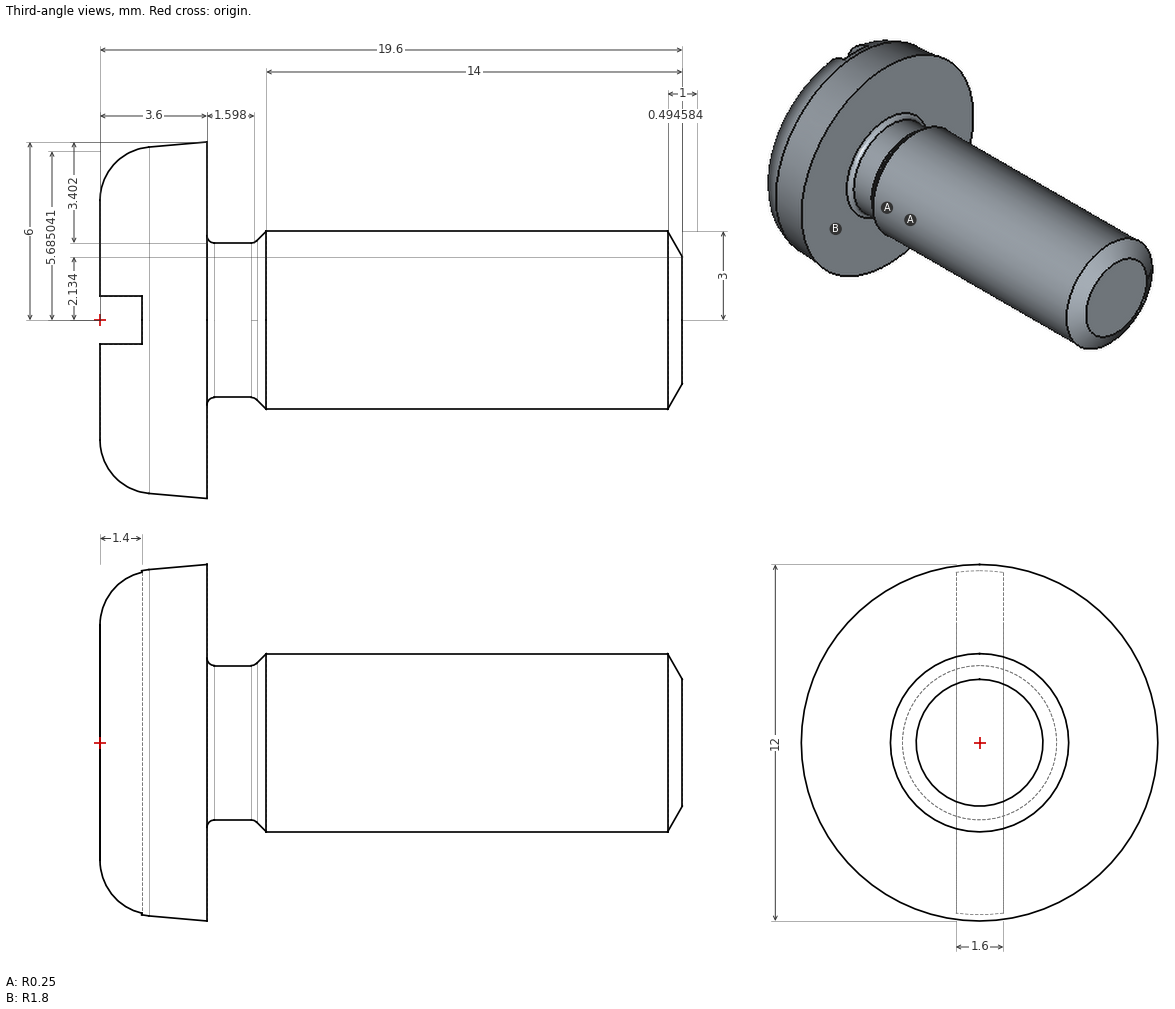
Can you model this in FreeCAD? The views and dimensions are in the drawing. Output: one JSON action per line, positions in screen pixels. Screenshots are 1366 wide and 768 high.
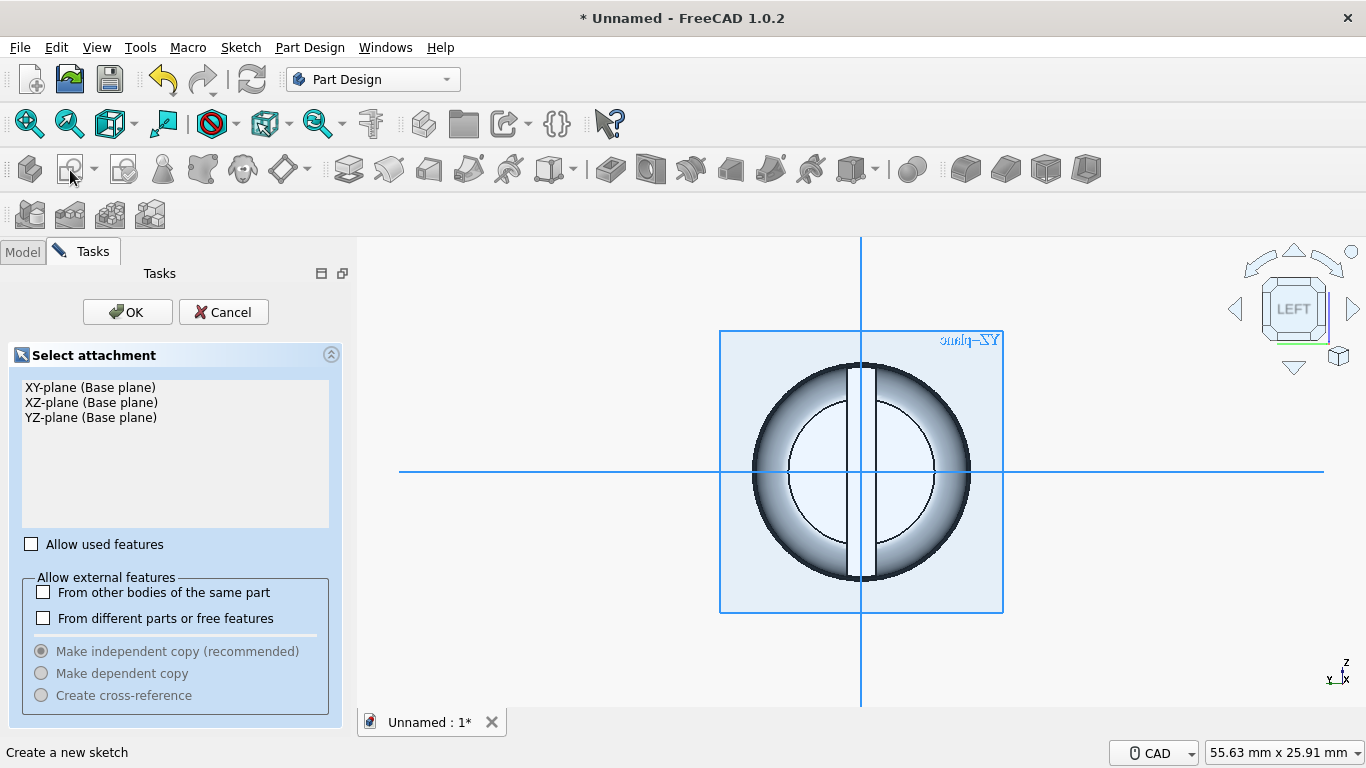
{"action": "left_click", "coordinate": [82, 388]}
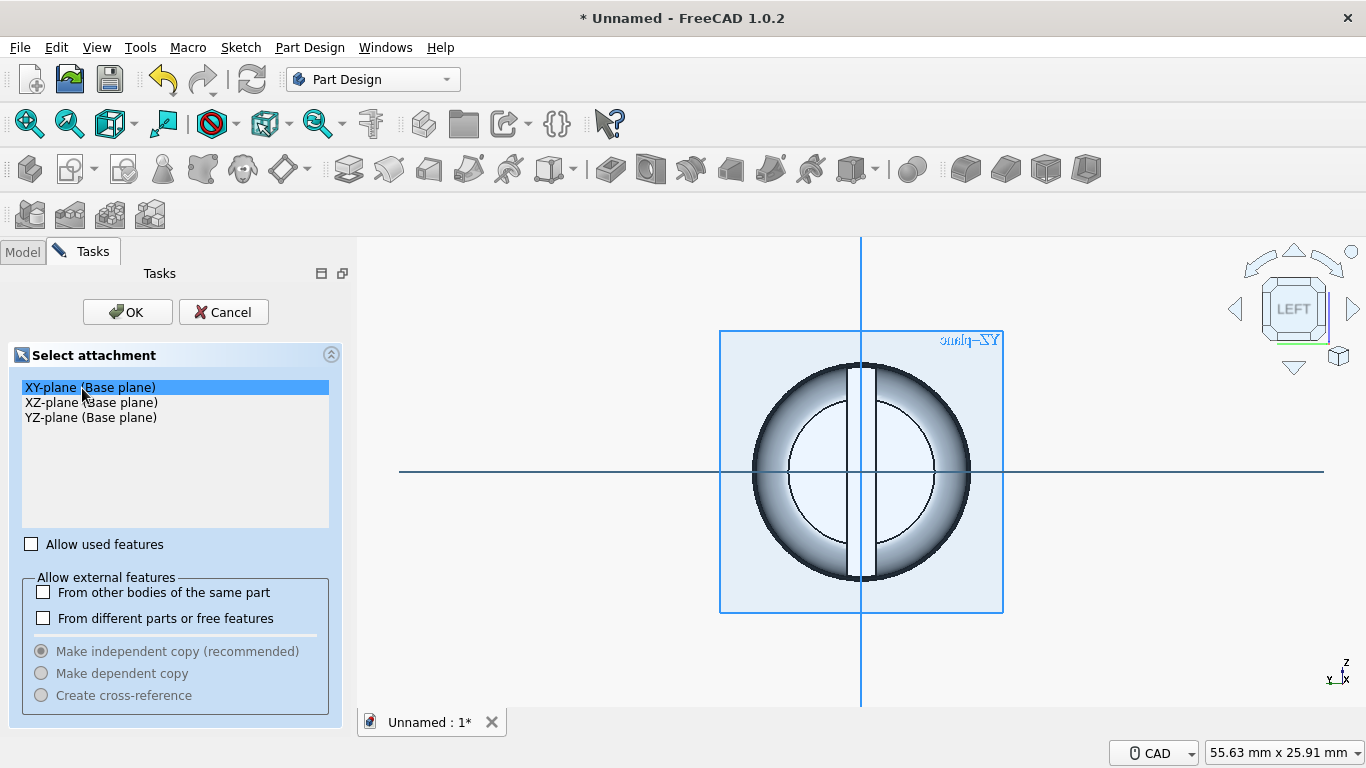
{"action": "left_click", "coordinate": [128, 312]}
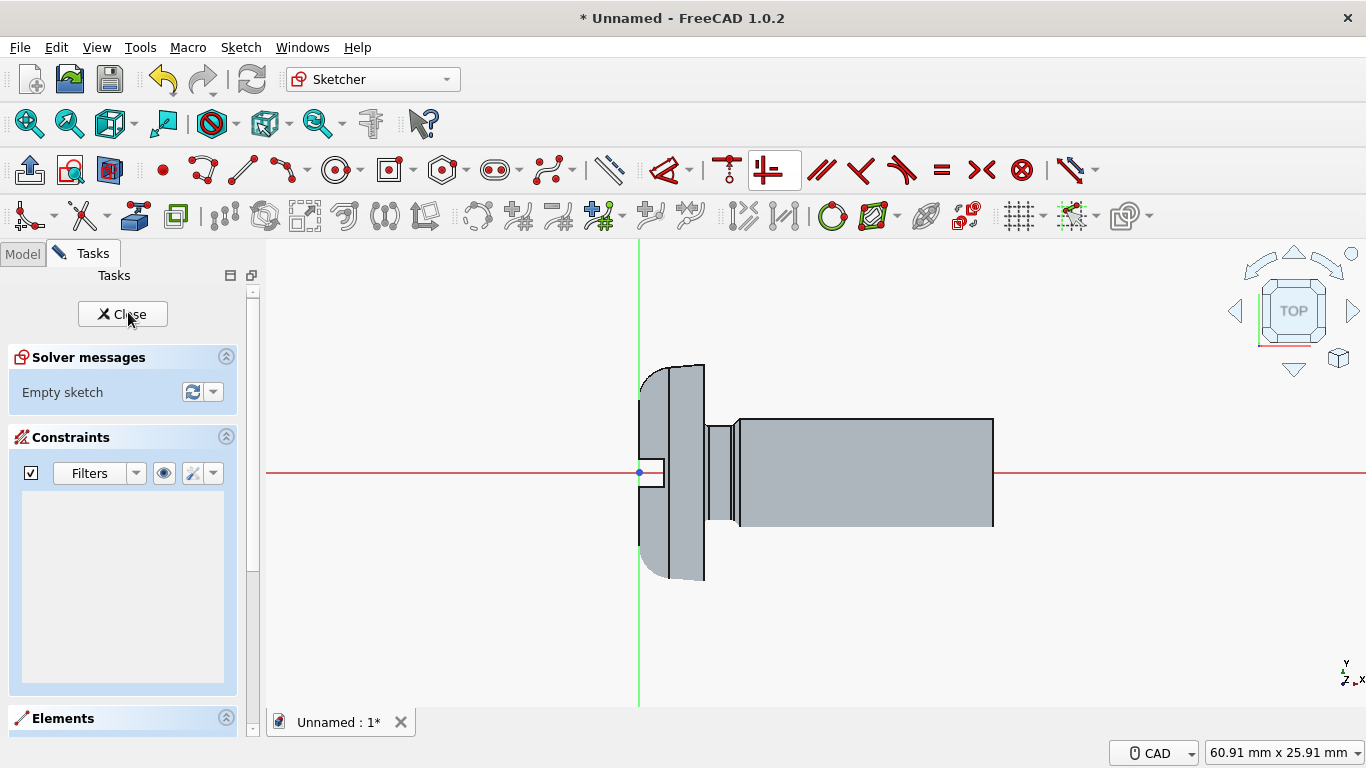
{"action": "left_click", "coordinate": [110, 170]}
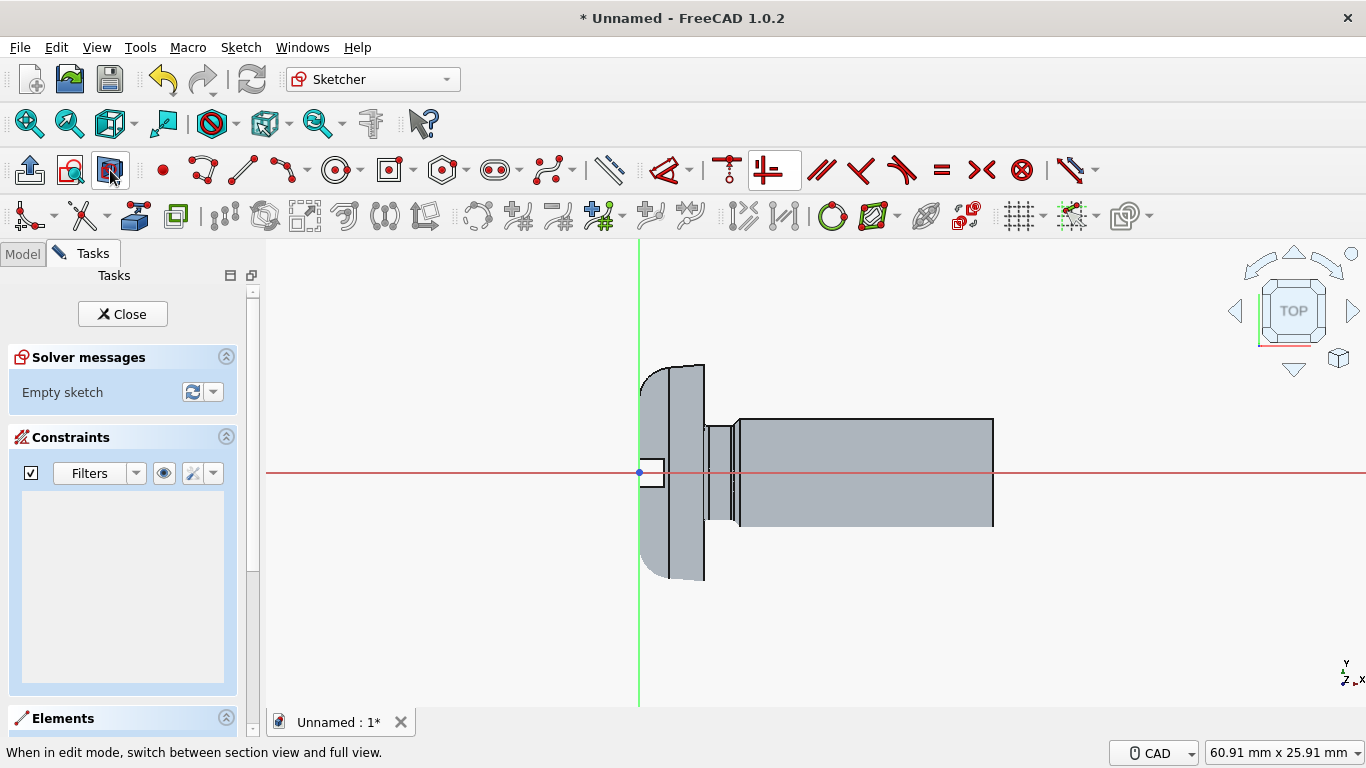
{"action": "scroll", "coordinate": [1006, 424], "scroll_direction": "up", "scroll_amount": 15}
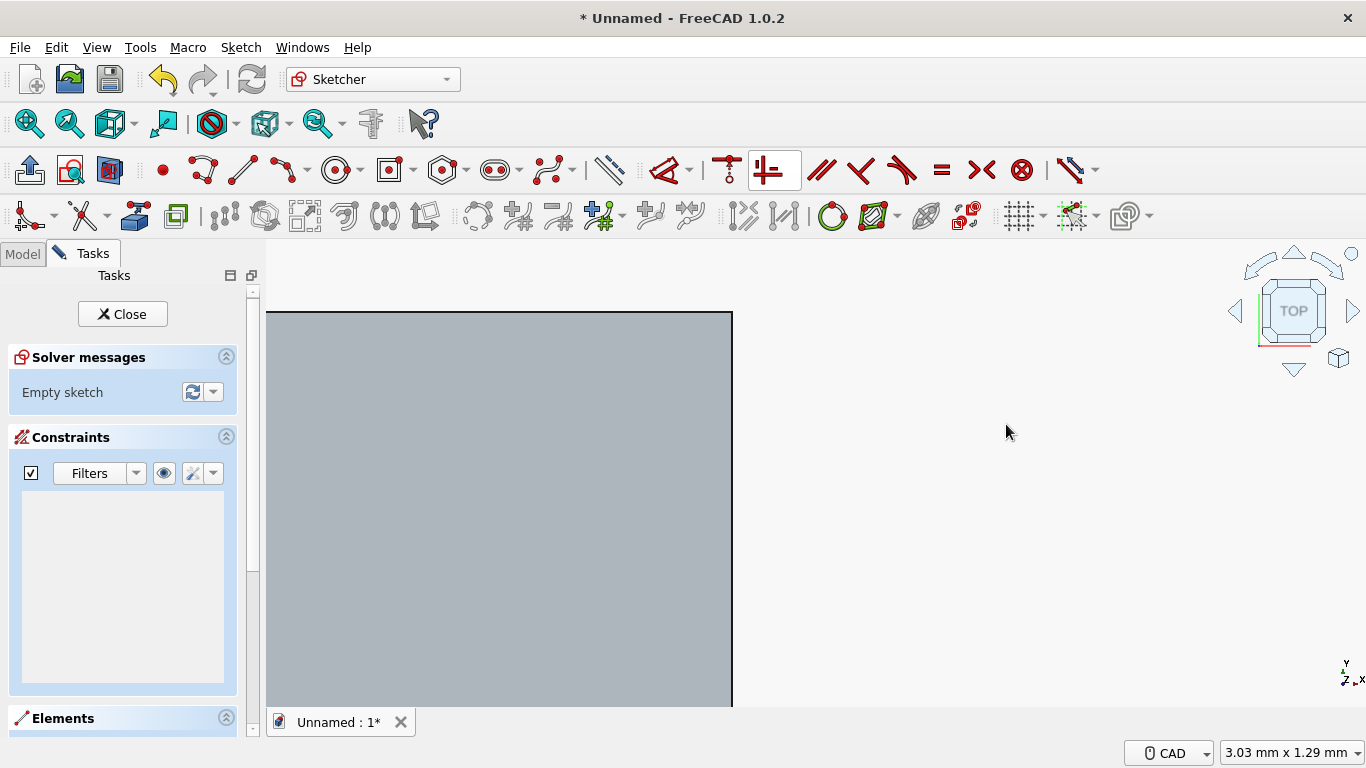
{"action": "left_click", "coordinate": [204, 170]}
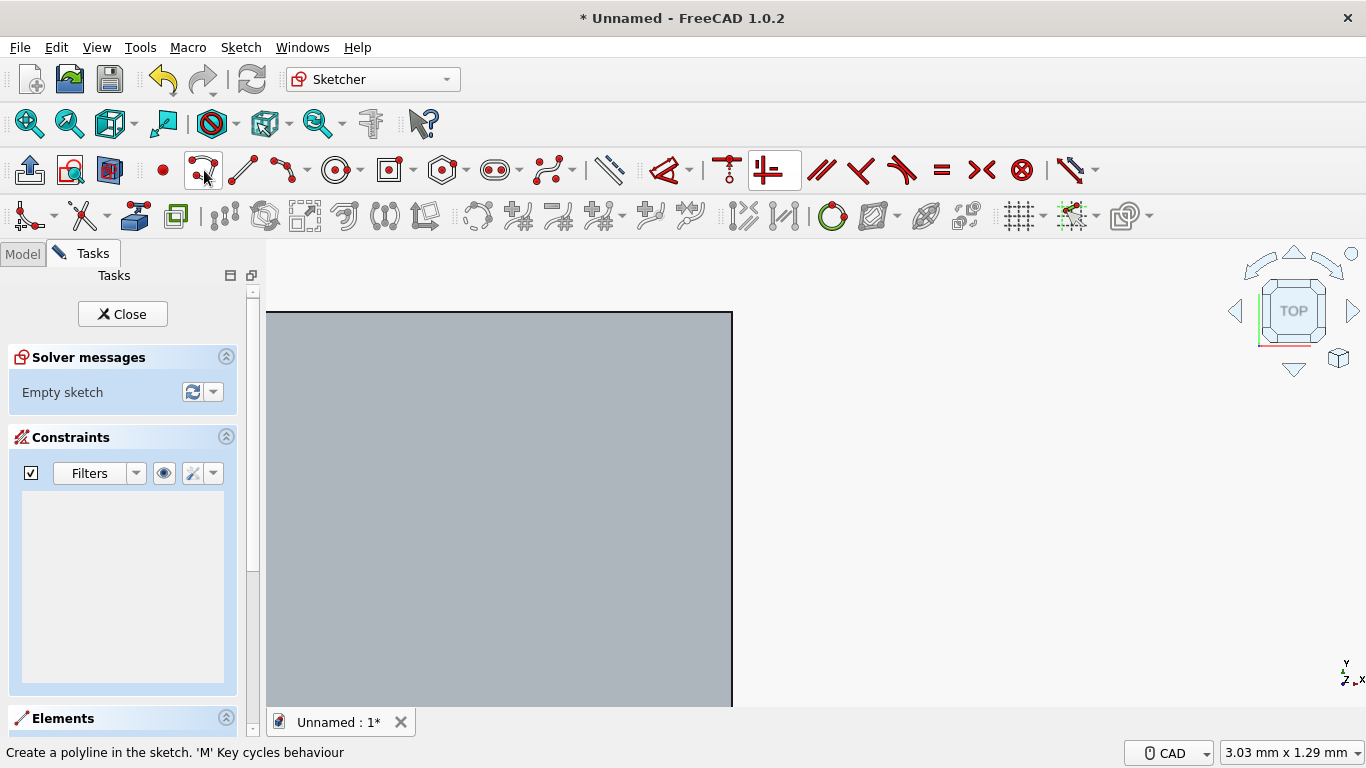
{"action": "left_click", "coordinate": [552, 312]}
{"action": "left_click", "coordinate": [732, 627]}
{"action": "left_click", "coordinate": [915, 312]}
{"action": "left_click", "coordinate": [552, 313]}
{"action": "key", "text": "Escape"}
{"action": "key", "text": "Escape"}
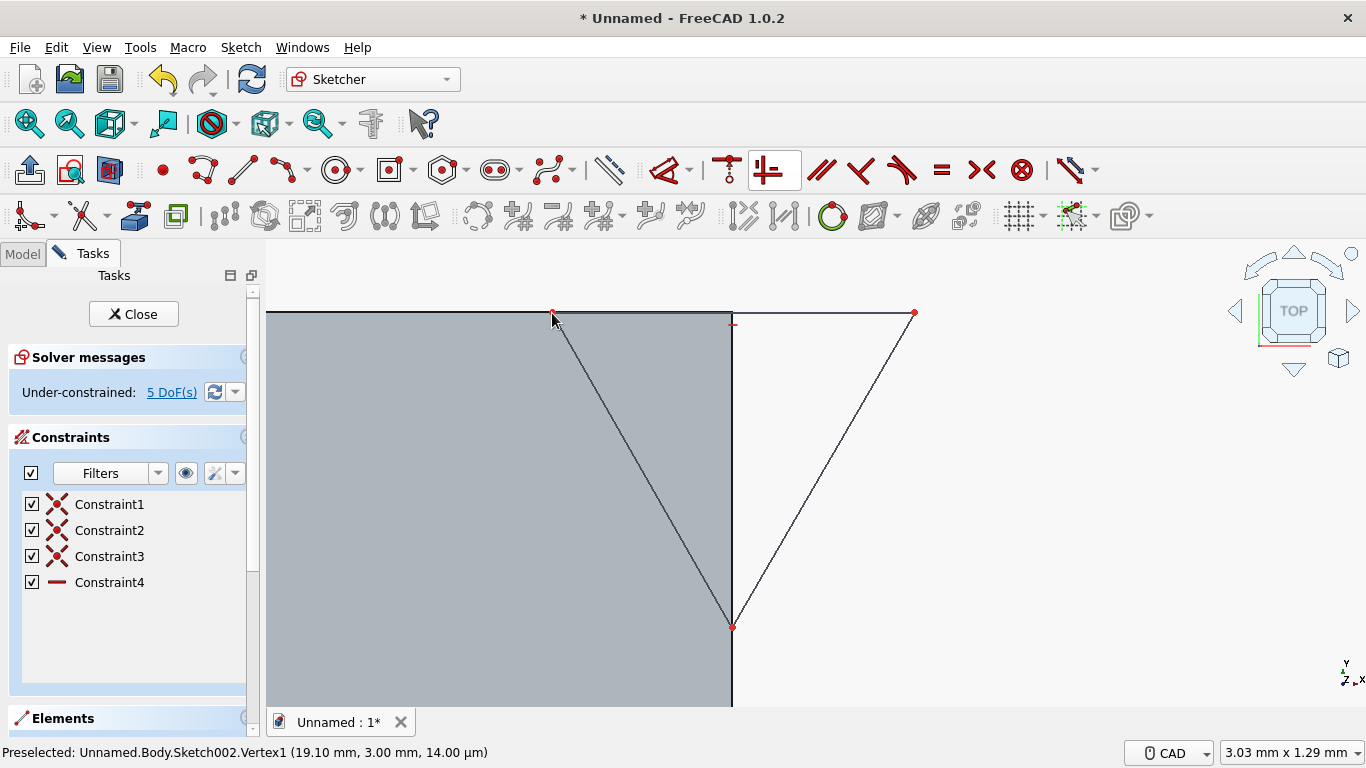
{"action": "left_click", "coordinate": [664, 170]}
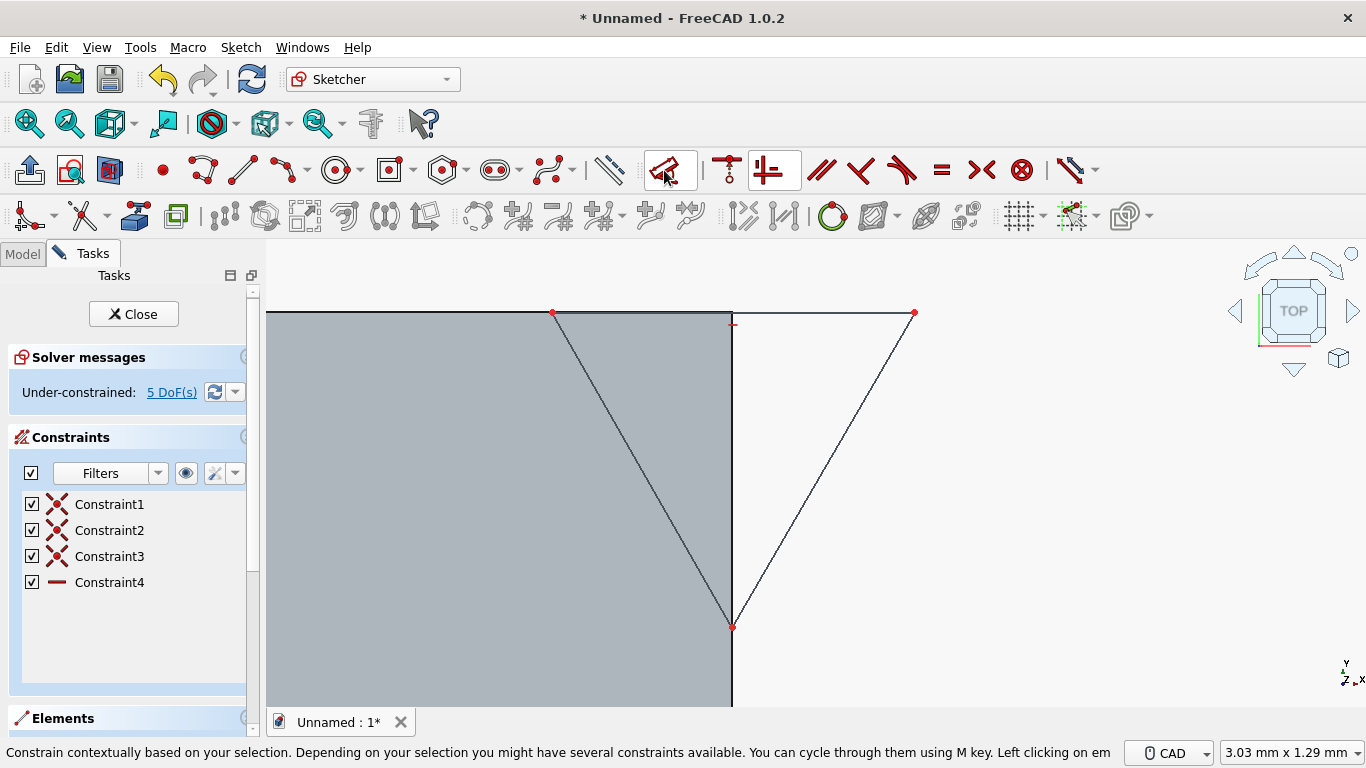
{"action": "left_click", "coordinate": [806, 313]}
{"action": "left_click", "coordinate": [733, 279]}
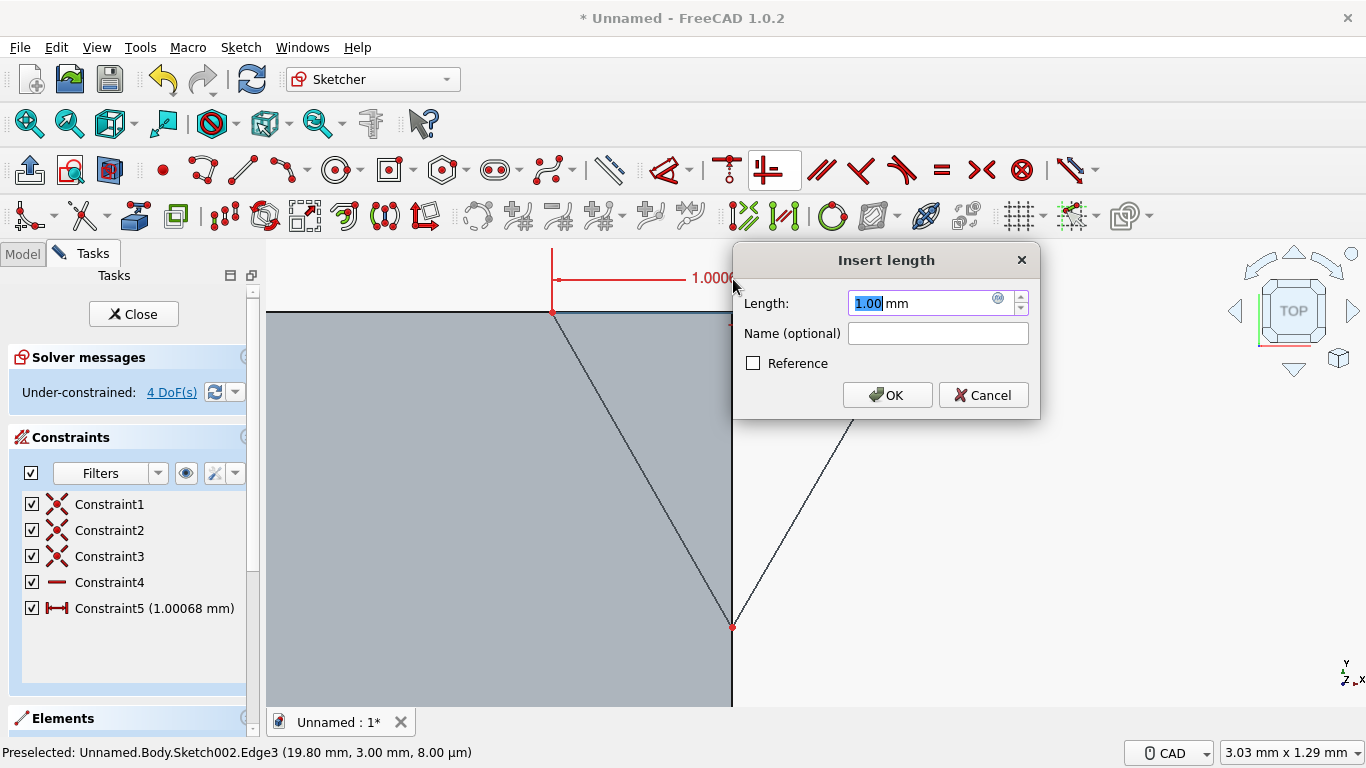
{"action": "type", "text": "1"}
{"action": "key", "text": "Return"}